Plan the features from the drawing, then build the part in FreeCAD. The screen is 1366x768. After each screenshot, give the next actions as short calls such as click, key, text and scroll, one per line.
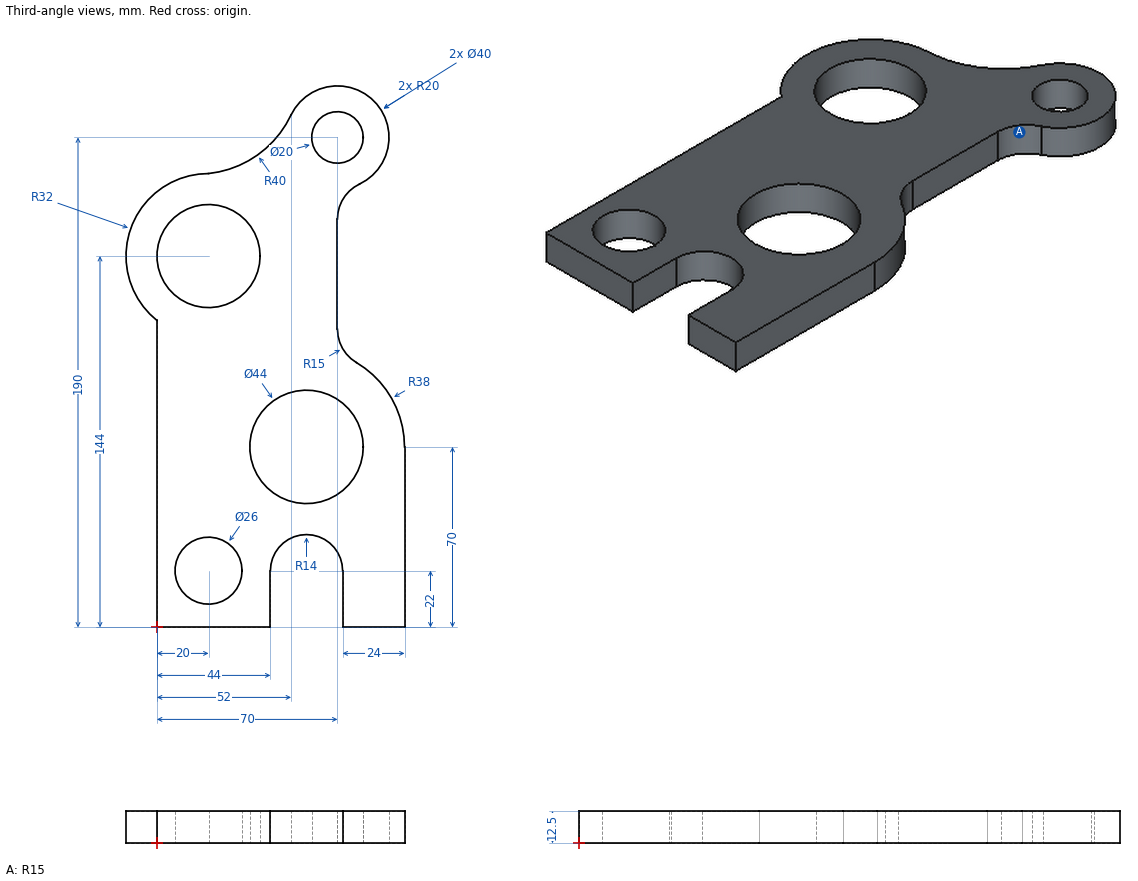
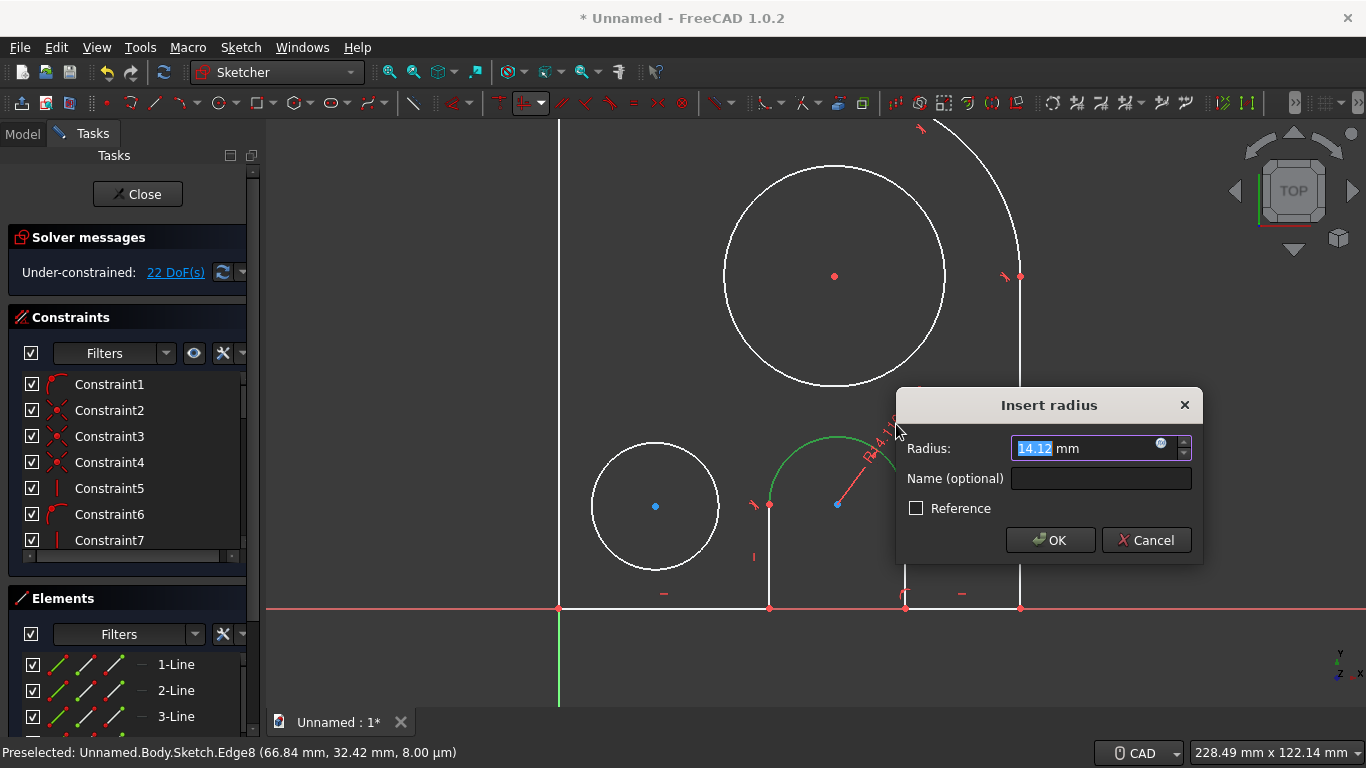
text(14)
key(Return)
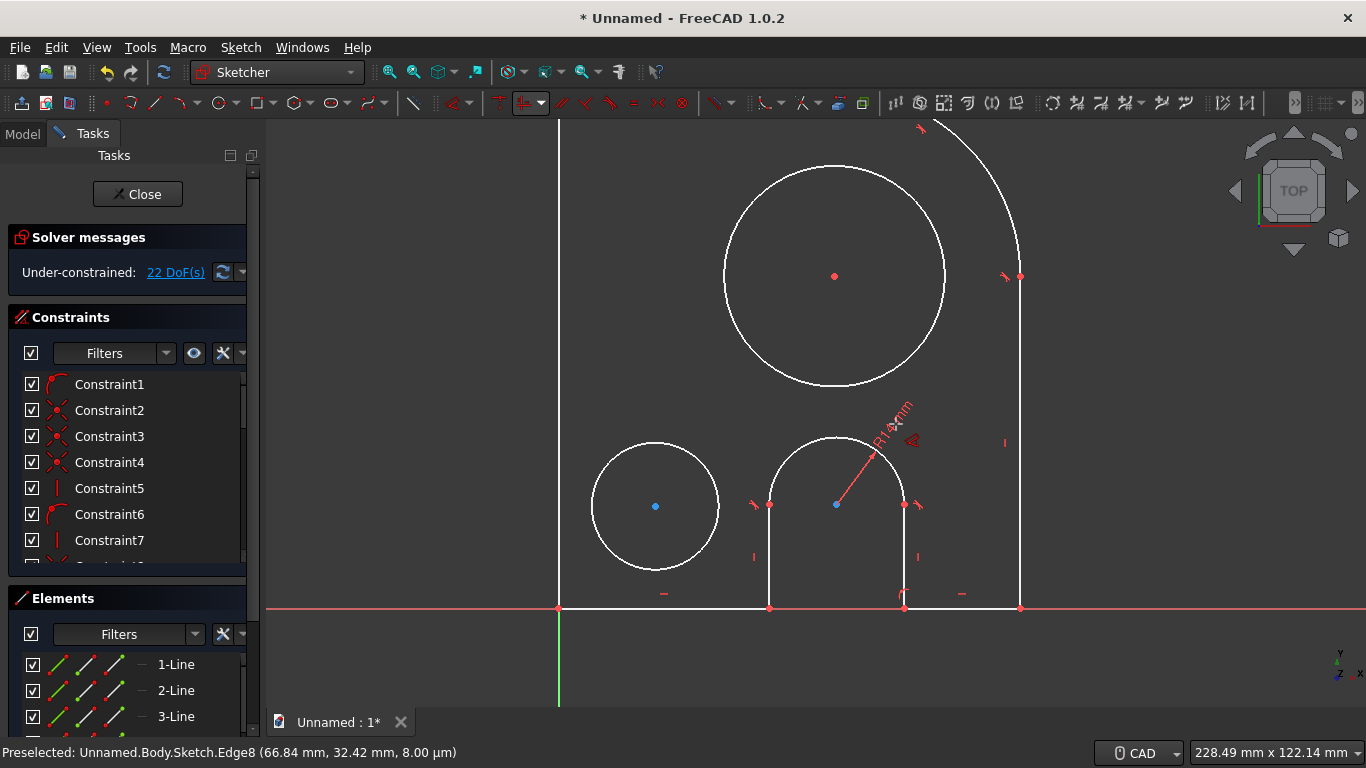
click(1011, 219)
click(1041, 209)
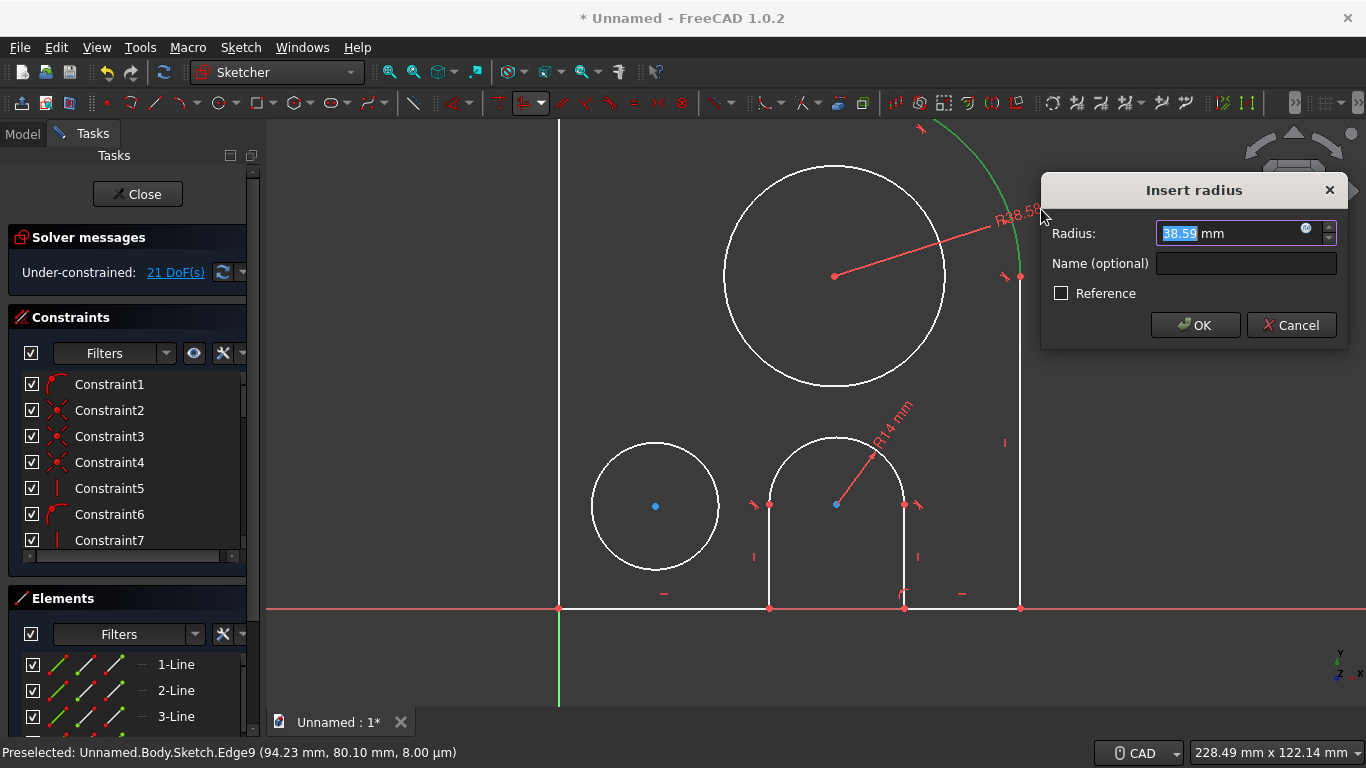
text(38)
key(Return)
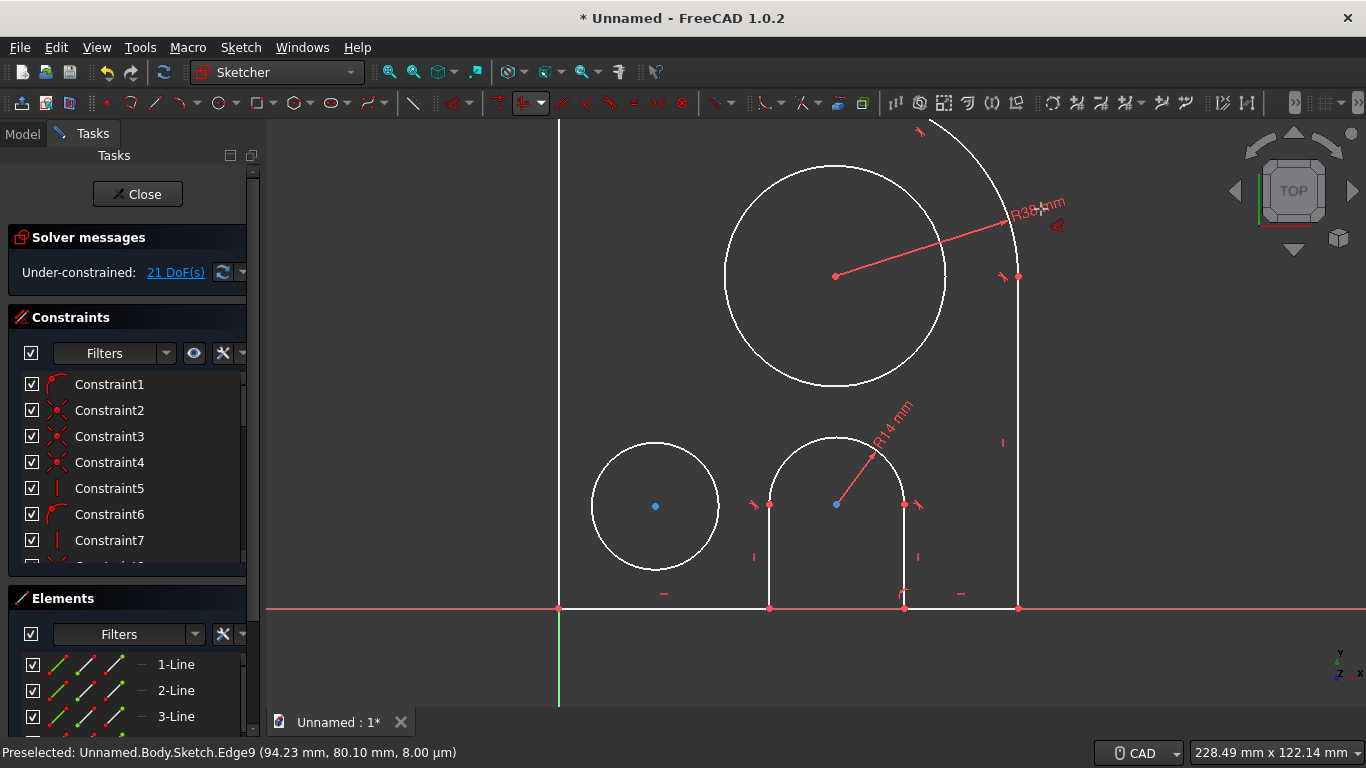
scroll(737, 580, down, 5)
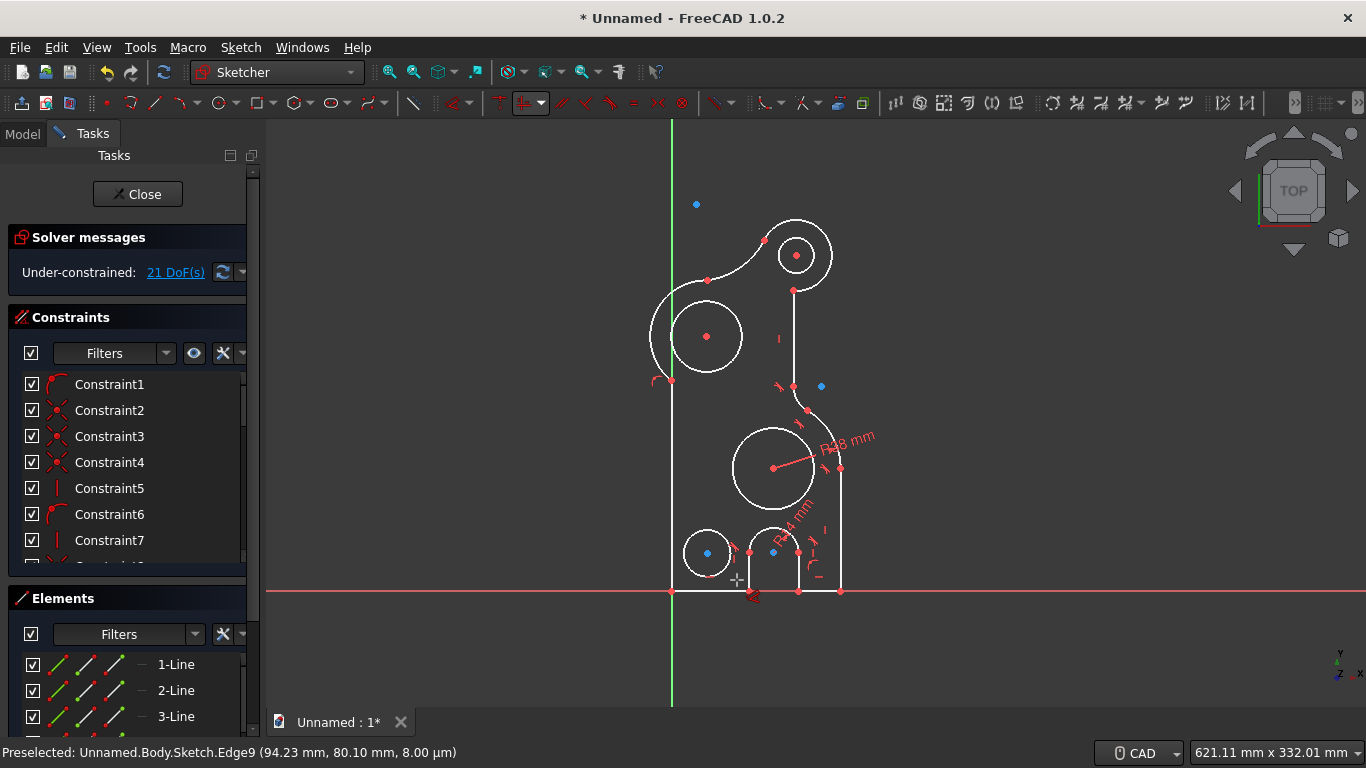
scroll(795, 395, up, 3)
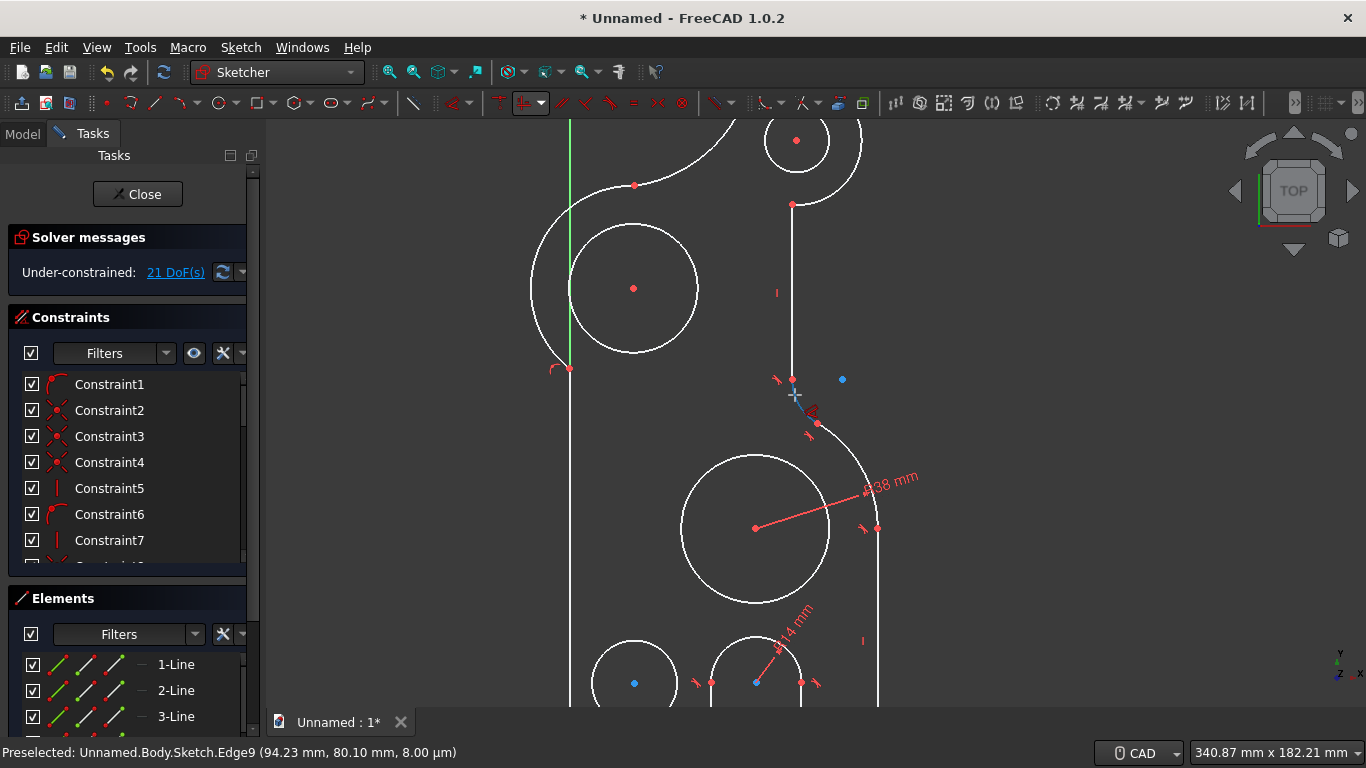
click(795, 395)
click(765, 405)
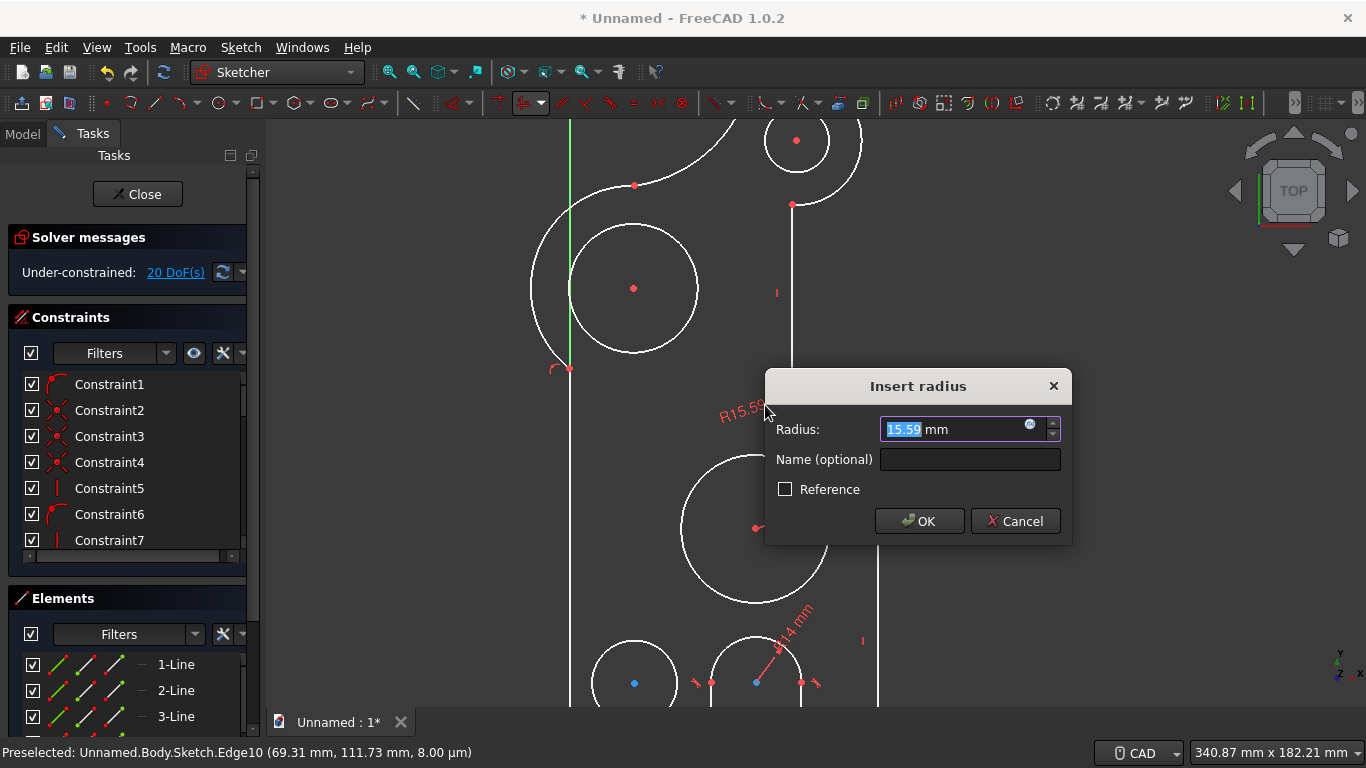
text(15)
key(Return)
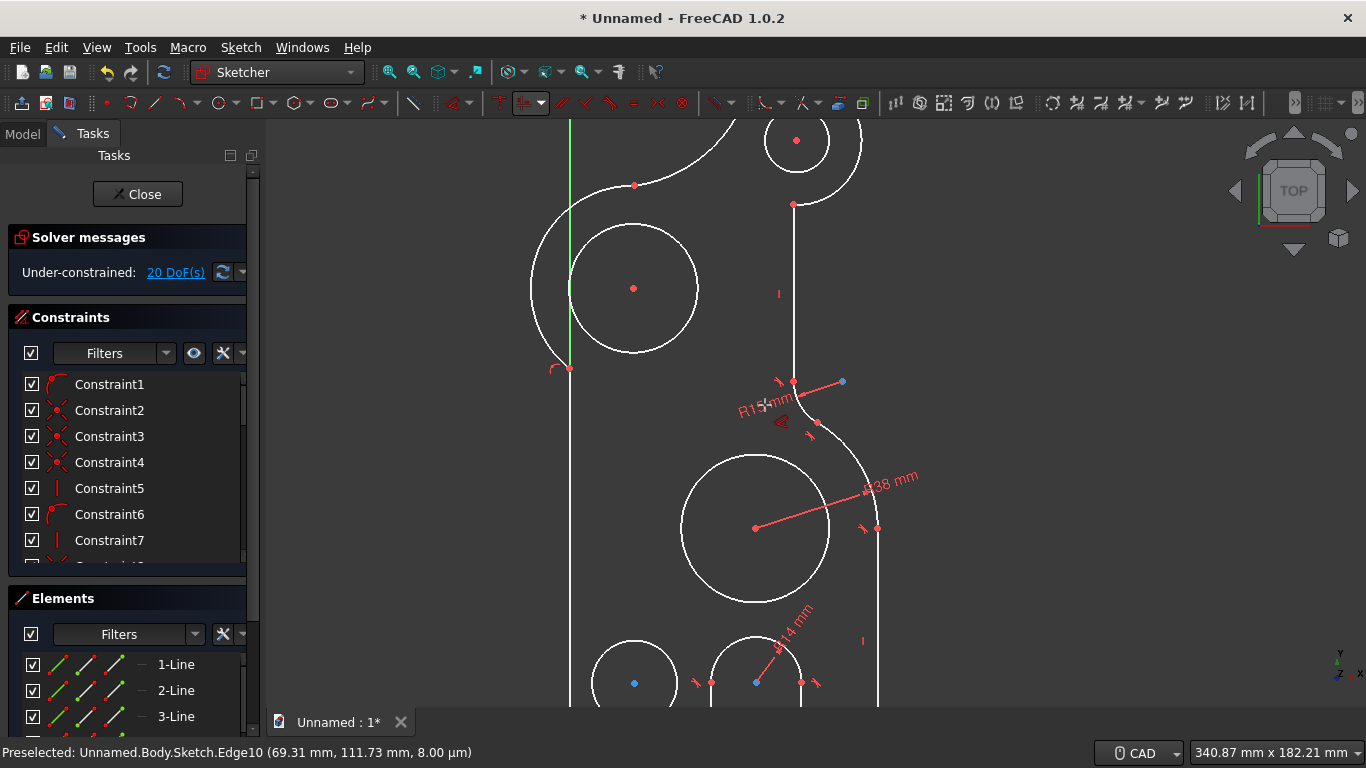
click(858, 161)
click(888, 171)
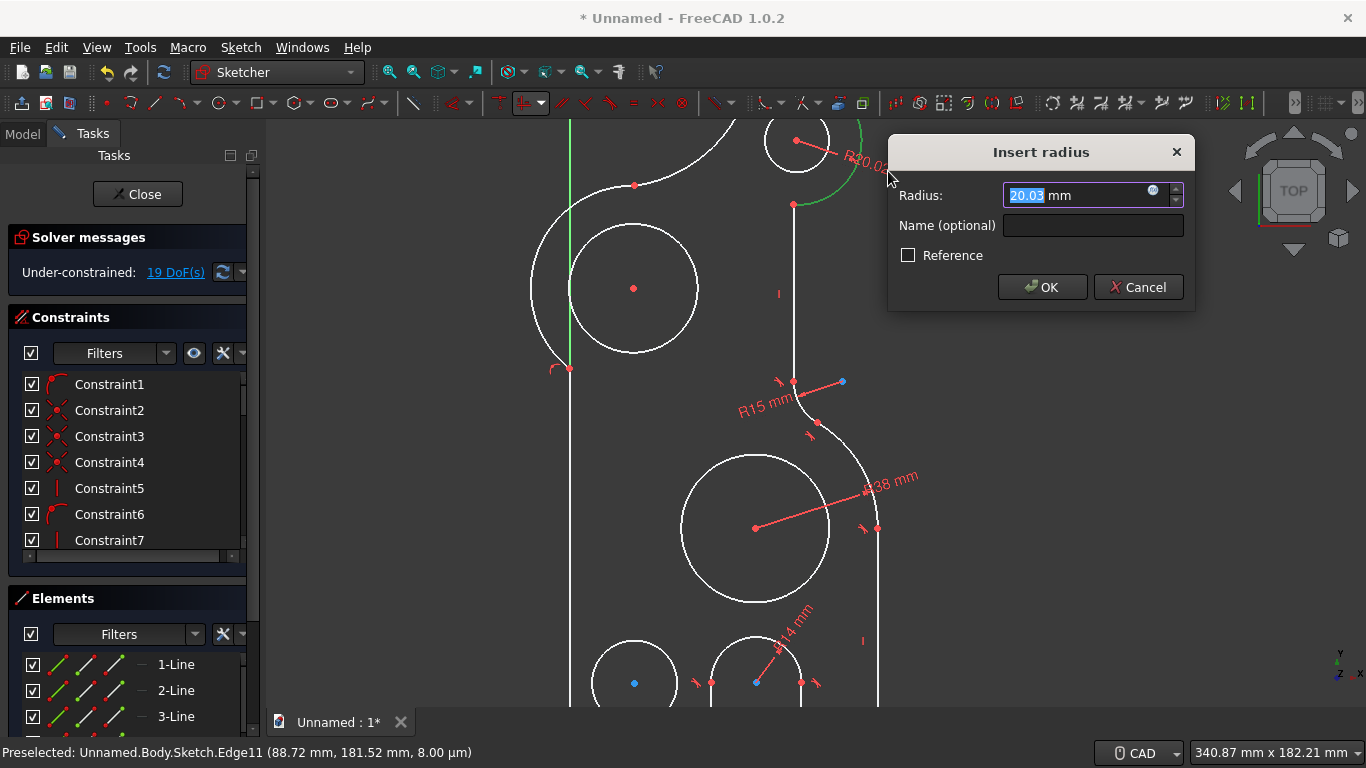
text(20)
key(Return)